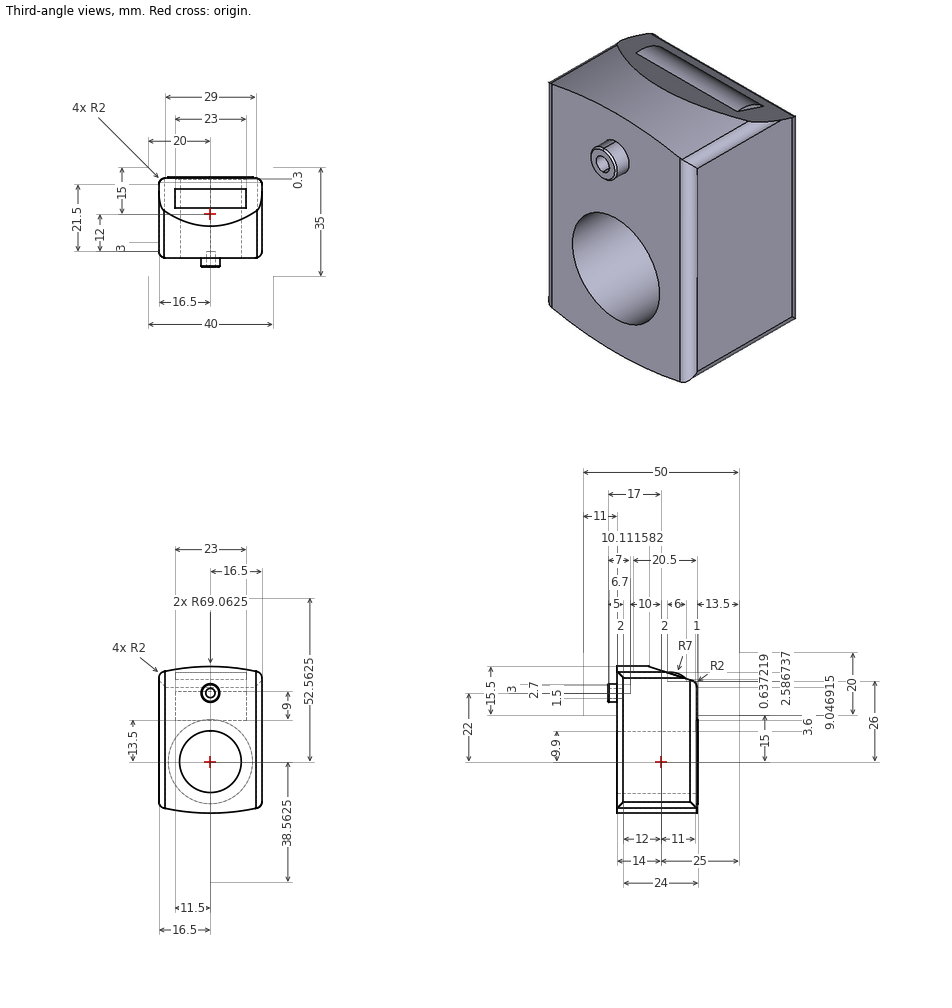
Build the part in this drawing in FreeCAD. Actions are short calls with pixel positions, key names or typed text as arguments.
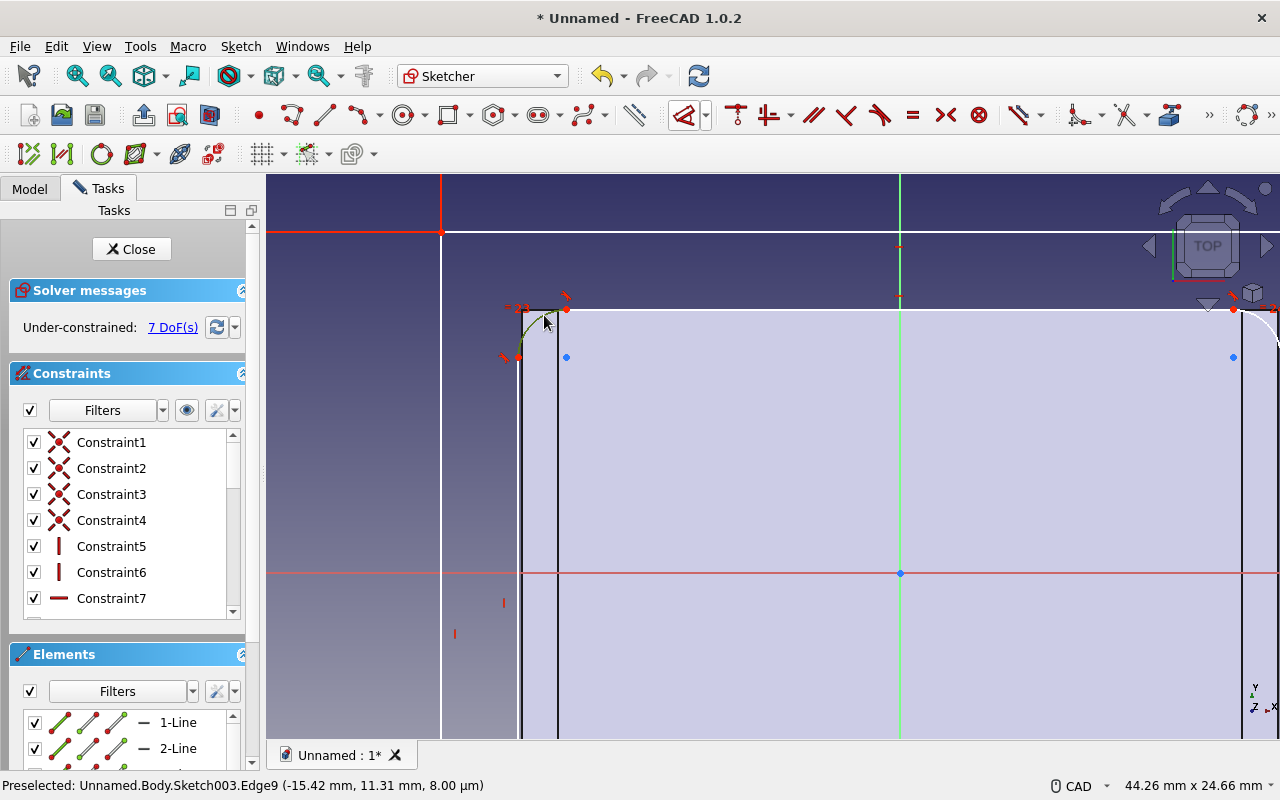
key(k)
key(r)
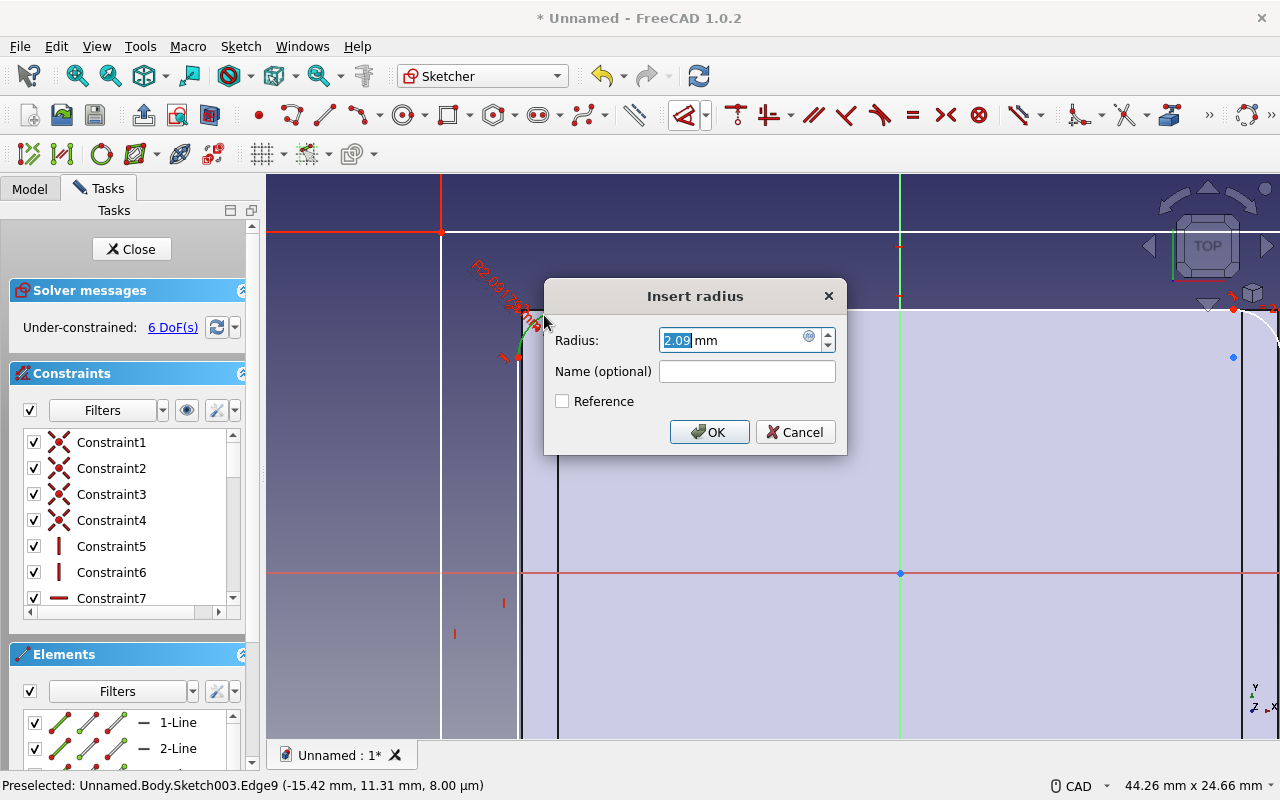
text(2)
key(Return)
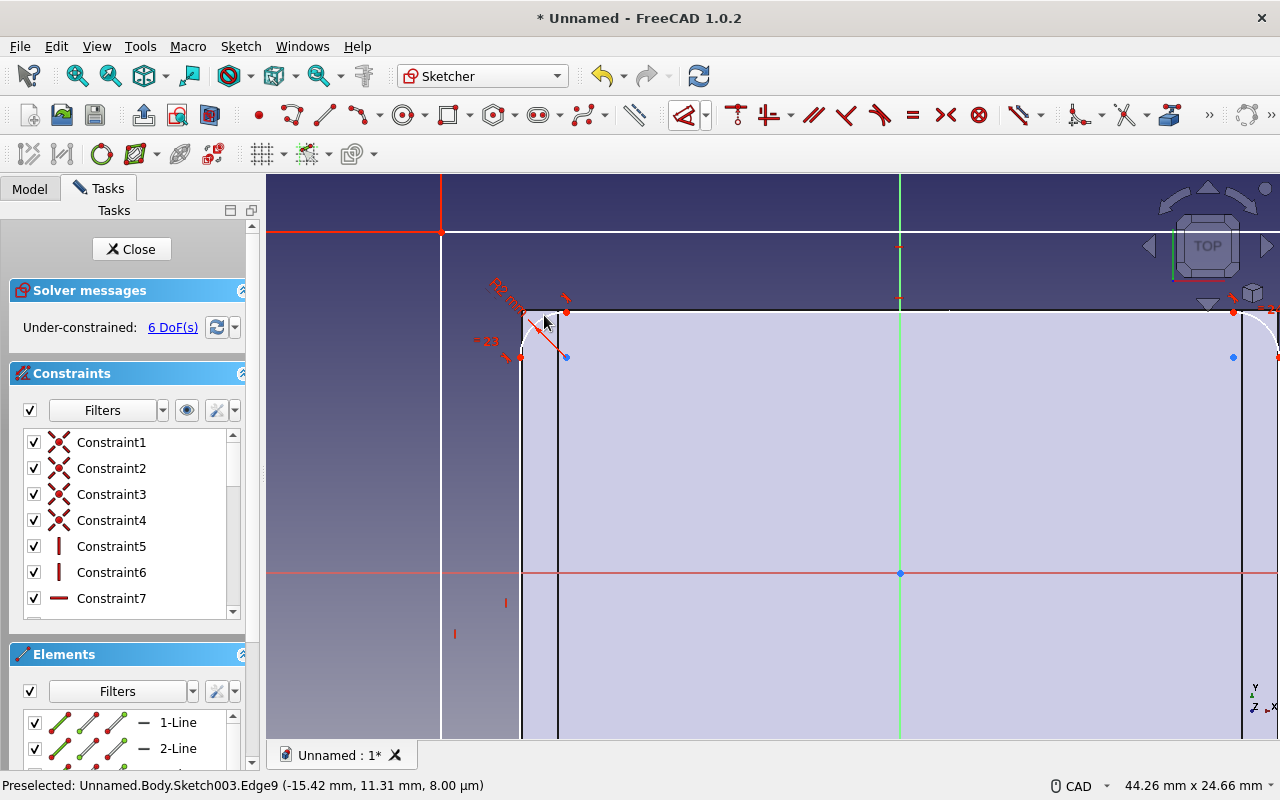
click(766, 312)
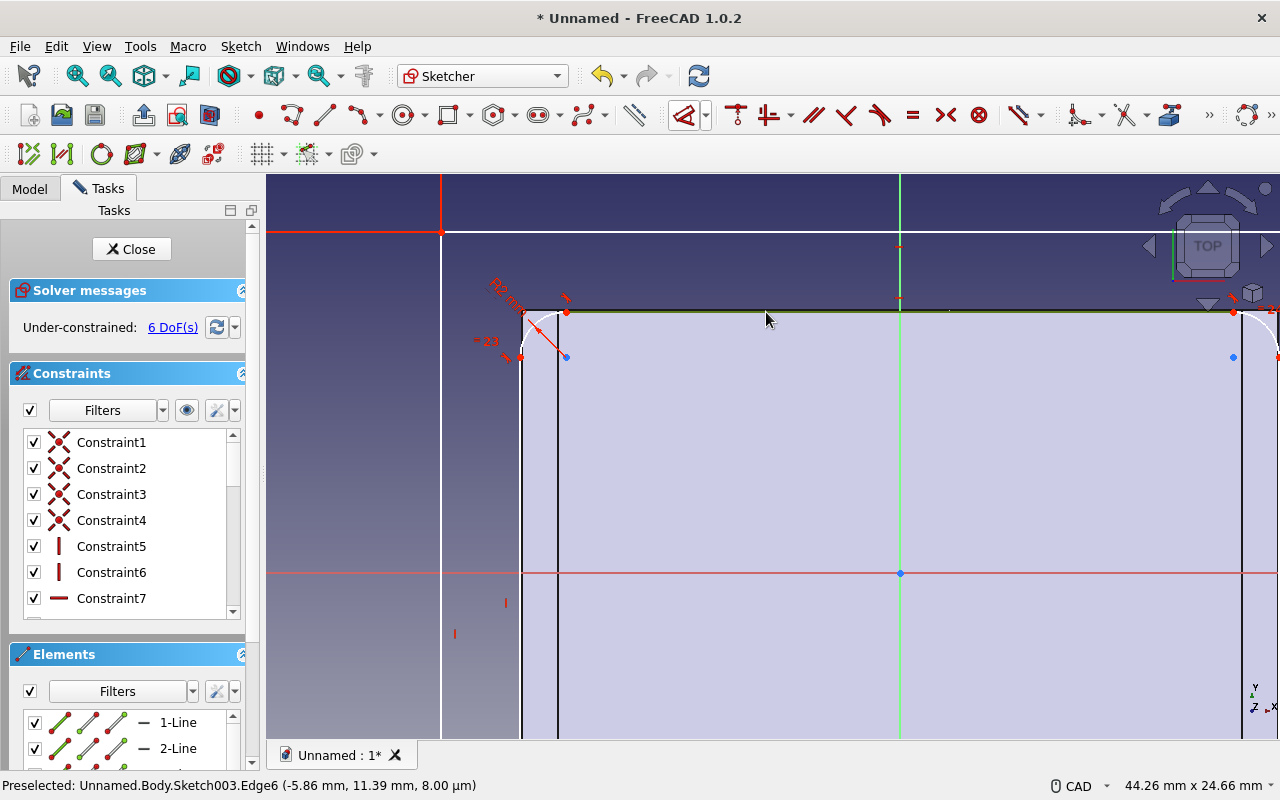
key(l)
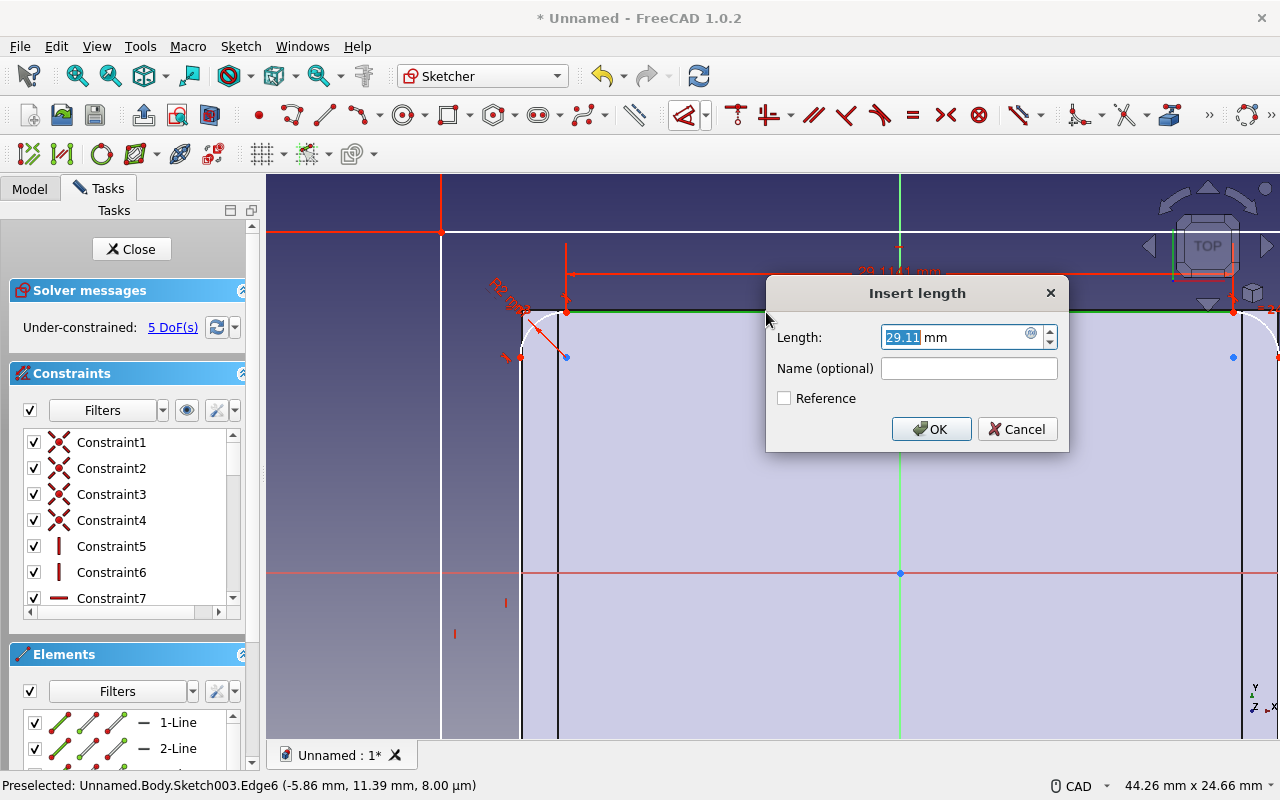
text(29)
key(Return)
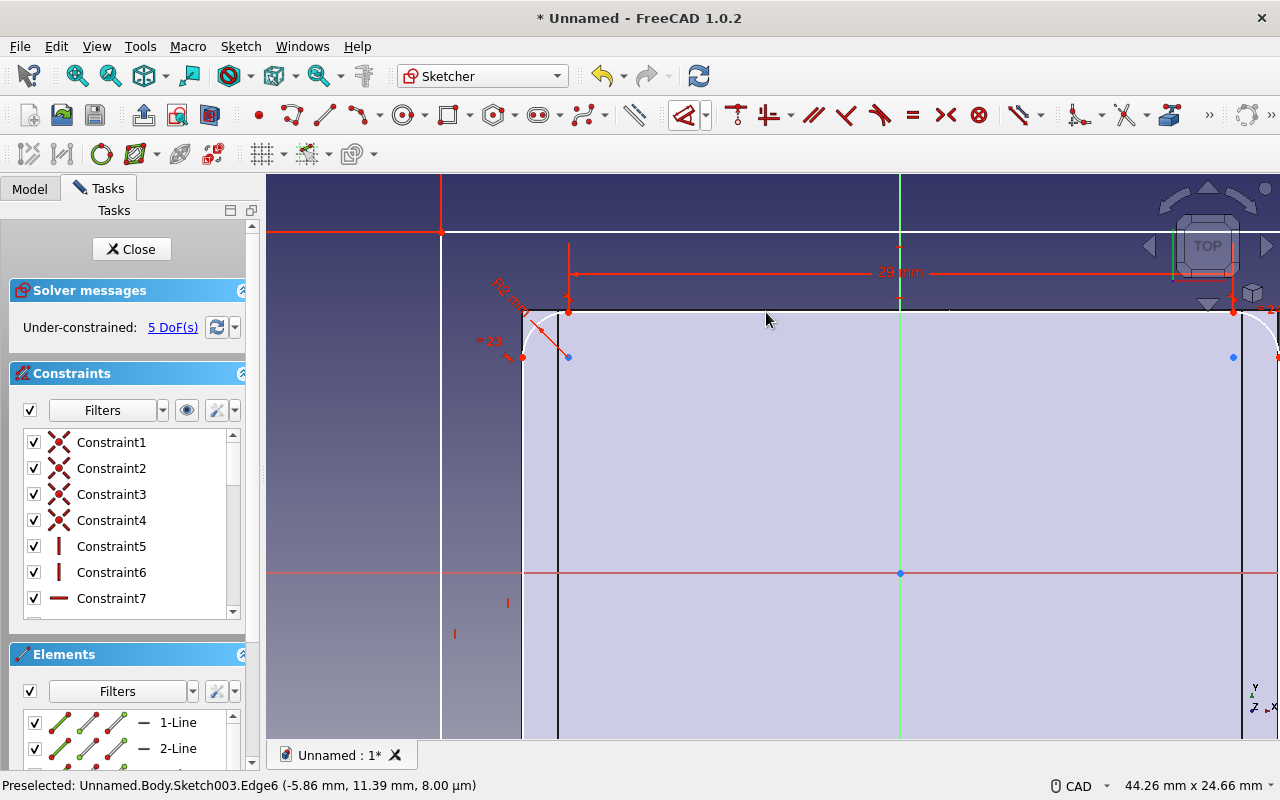
click(441, 232)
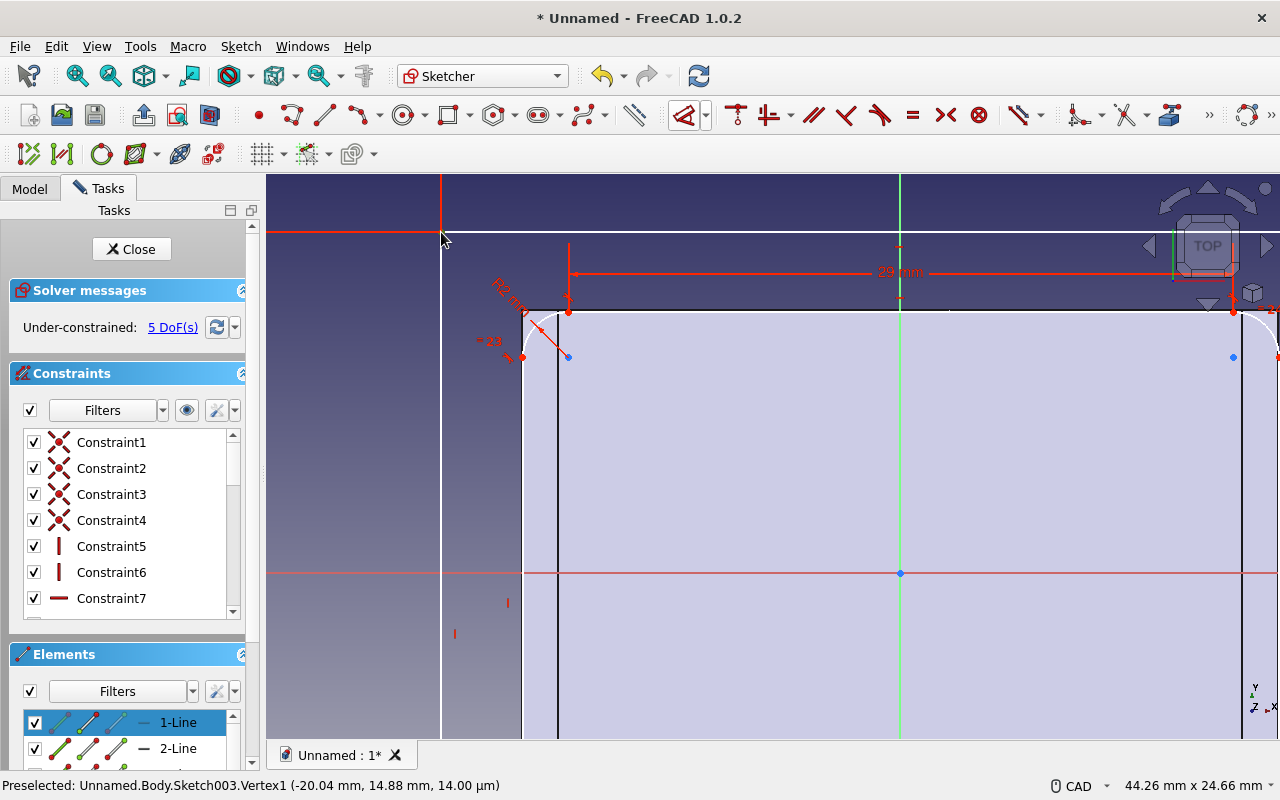
click(706, 116)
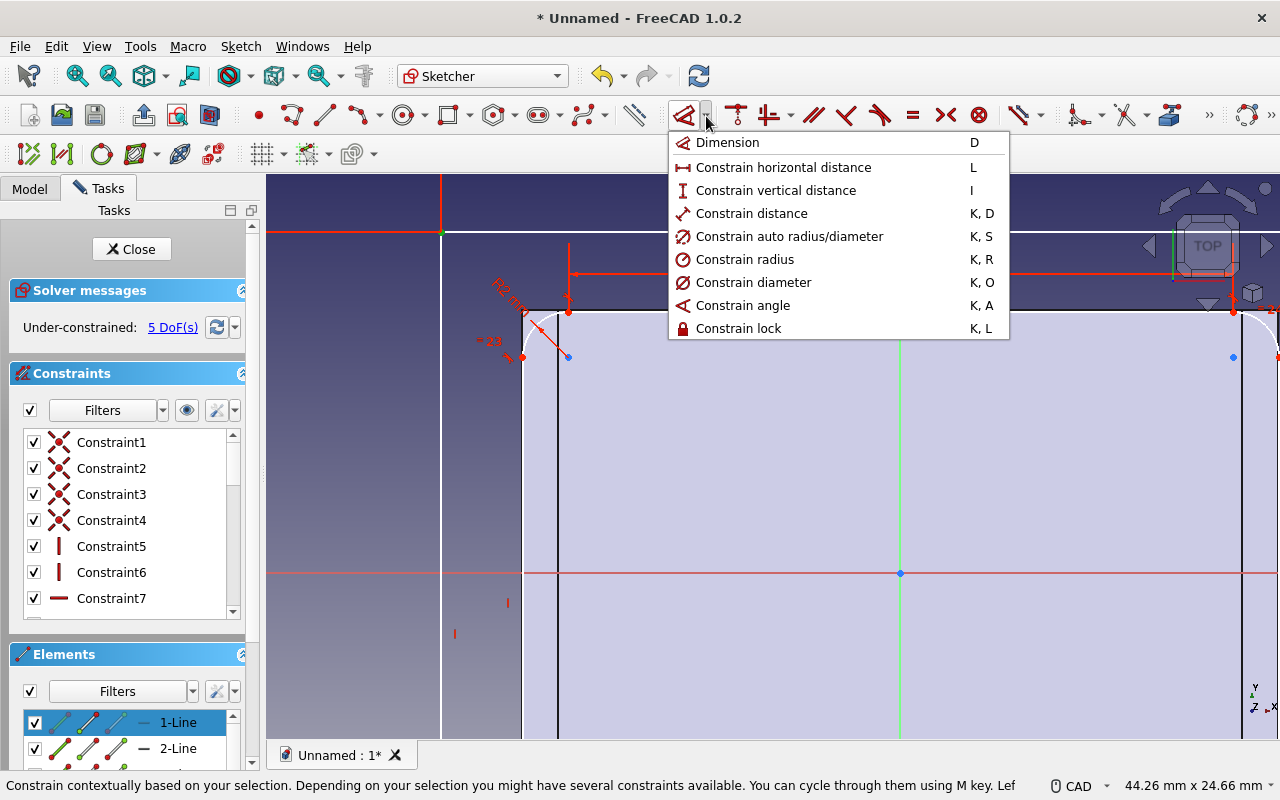
click(839, 168)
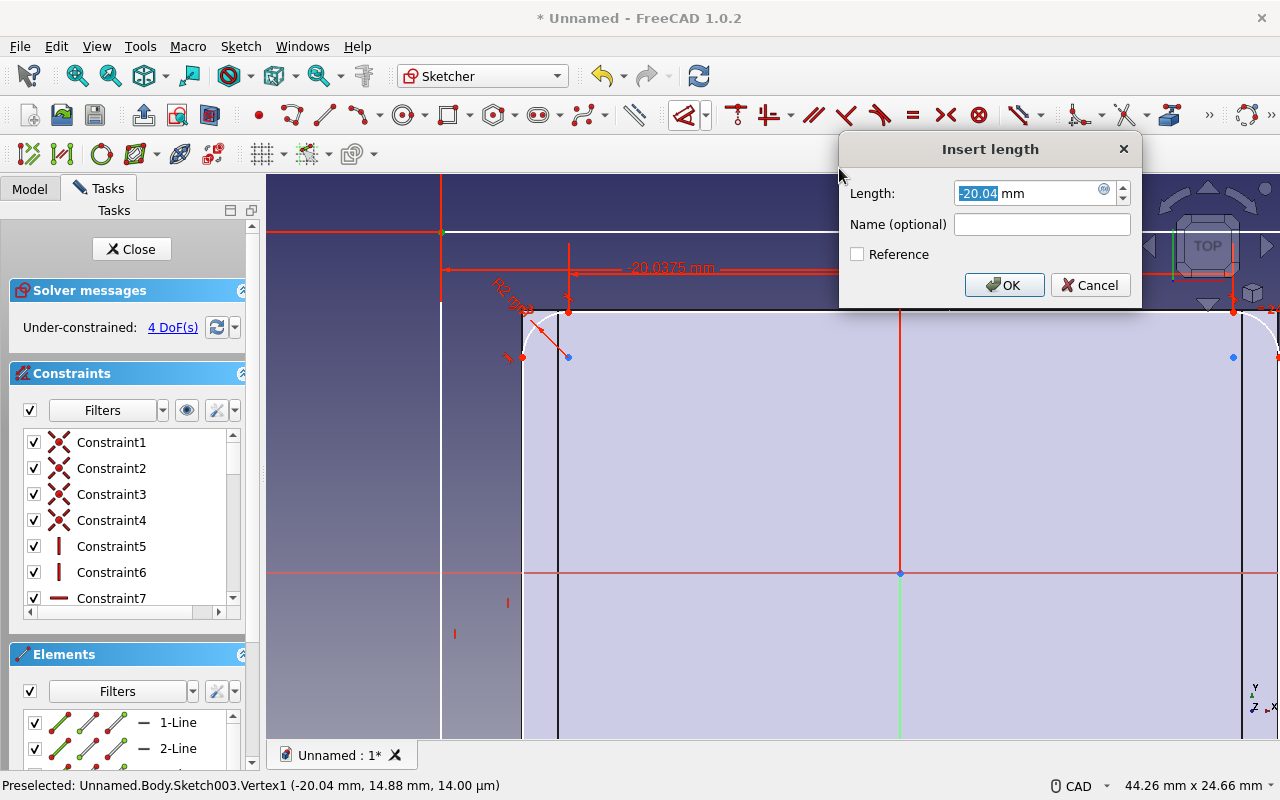
text(-20)
key(Return)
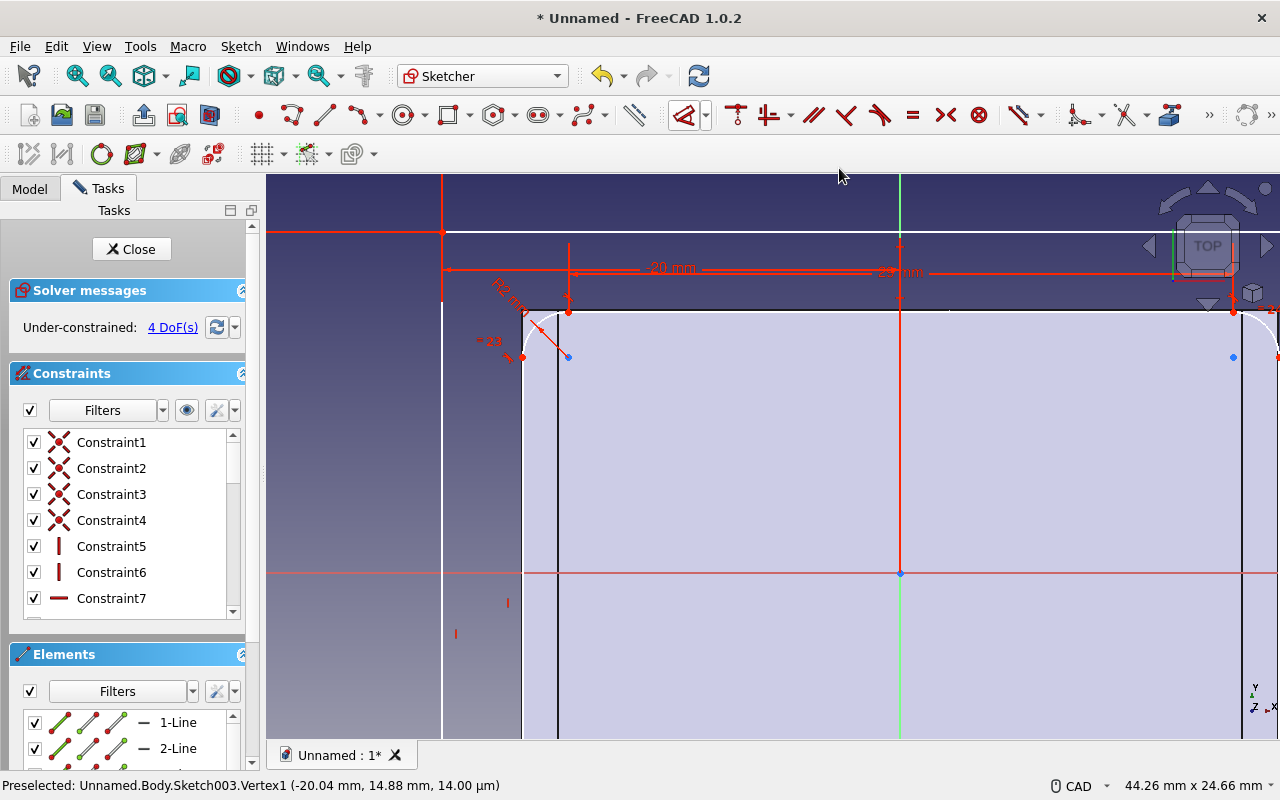
click(442, 232)